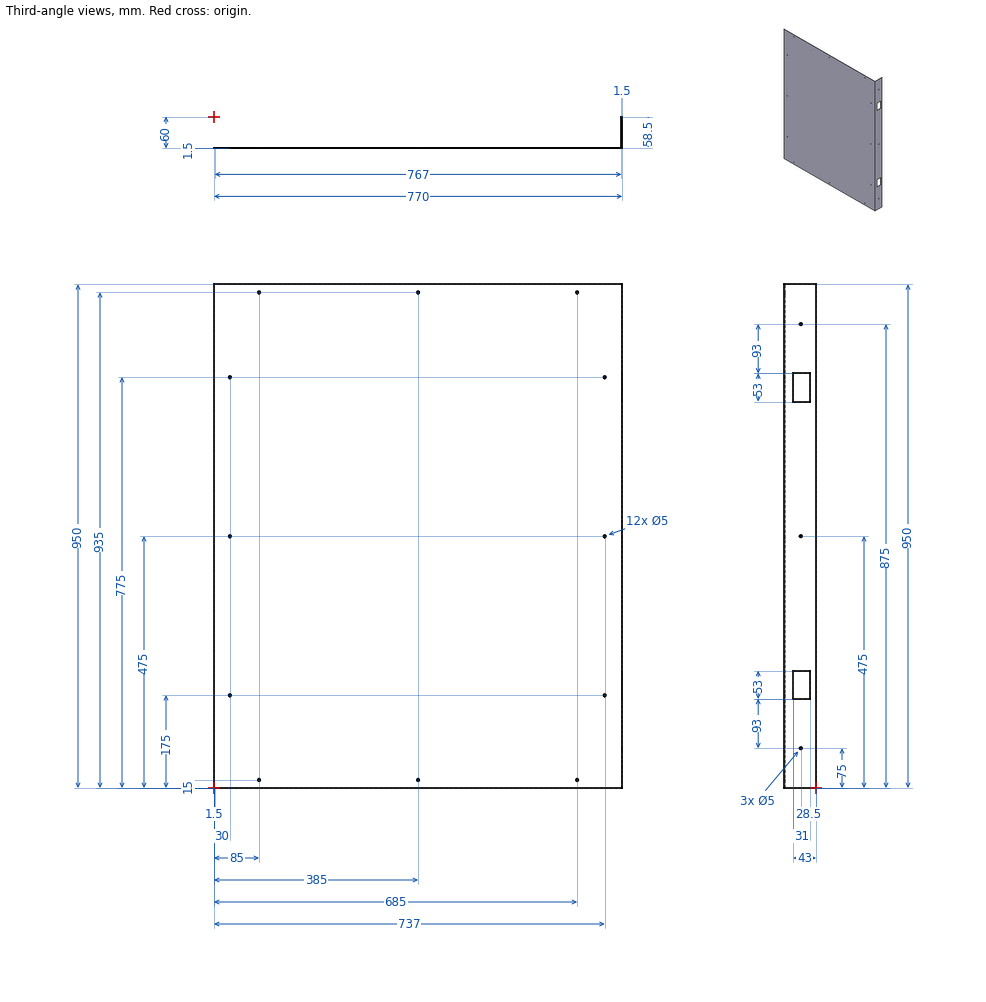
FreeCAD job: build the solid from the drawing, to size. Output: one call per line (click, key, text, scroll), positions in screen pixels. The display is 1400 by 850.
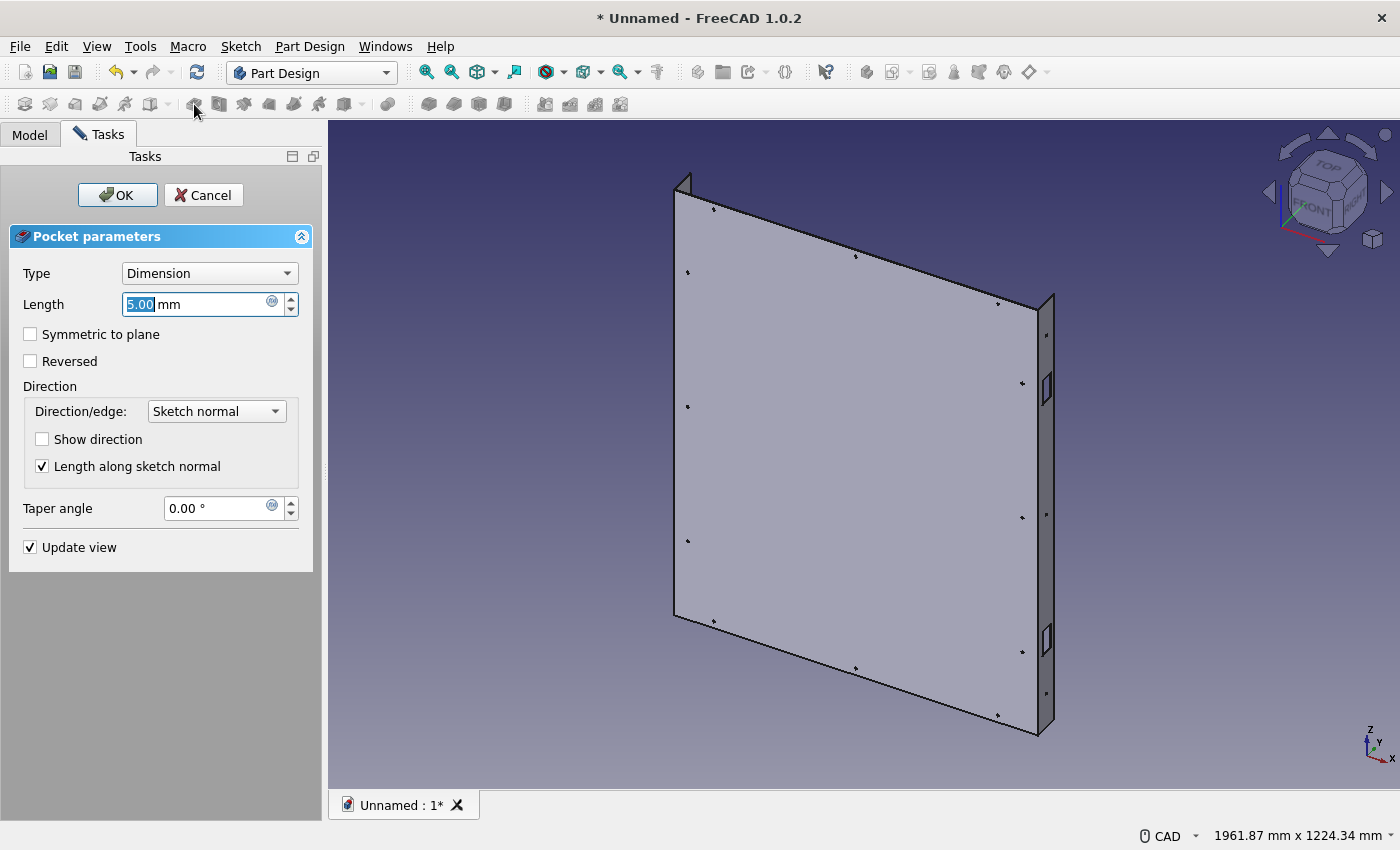
text(1.5)
key(Tab)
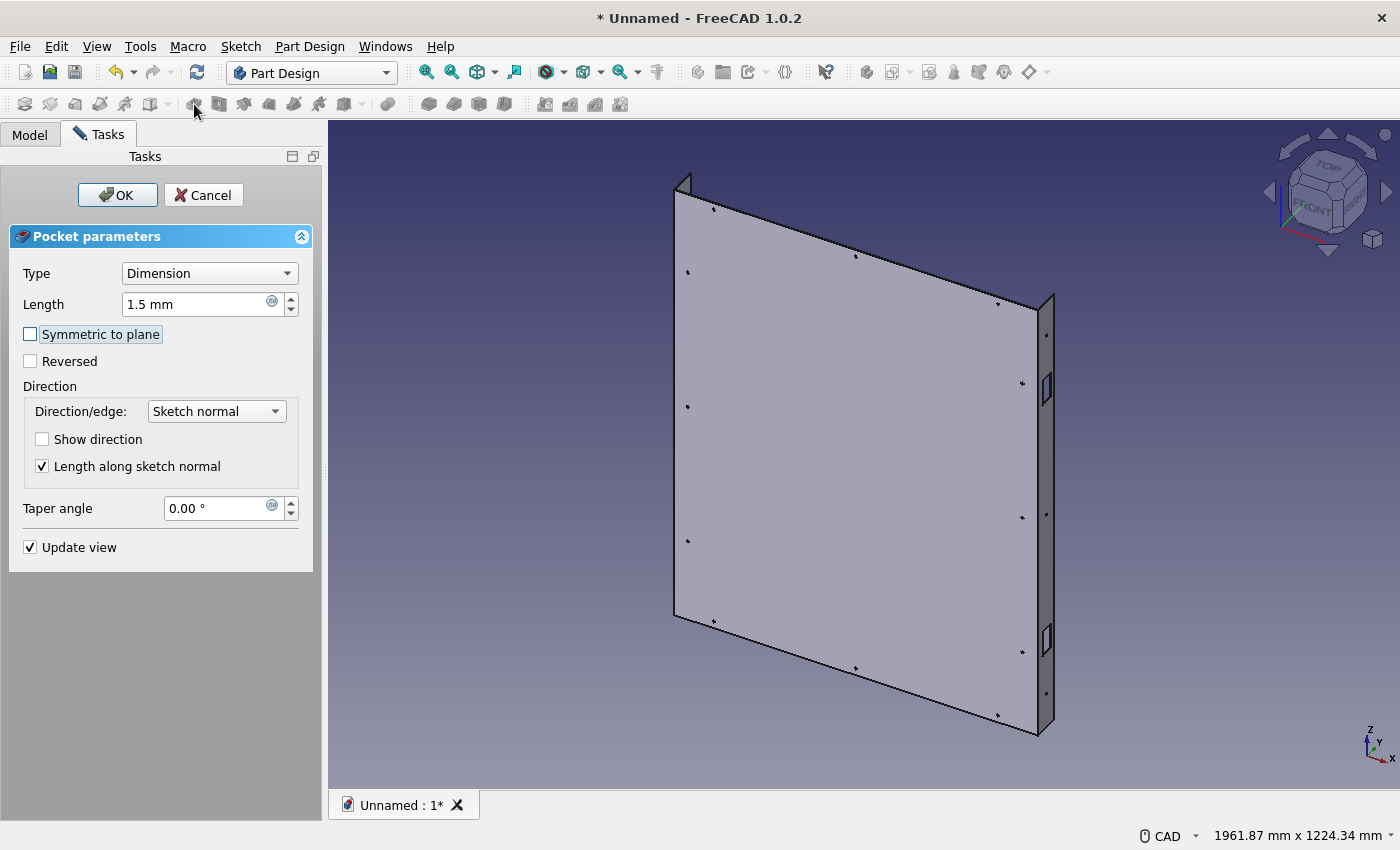
click(118, 195)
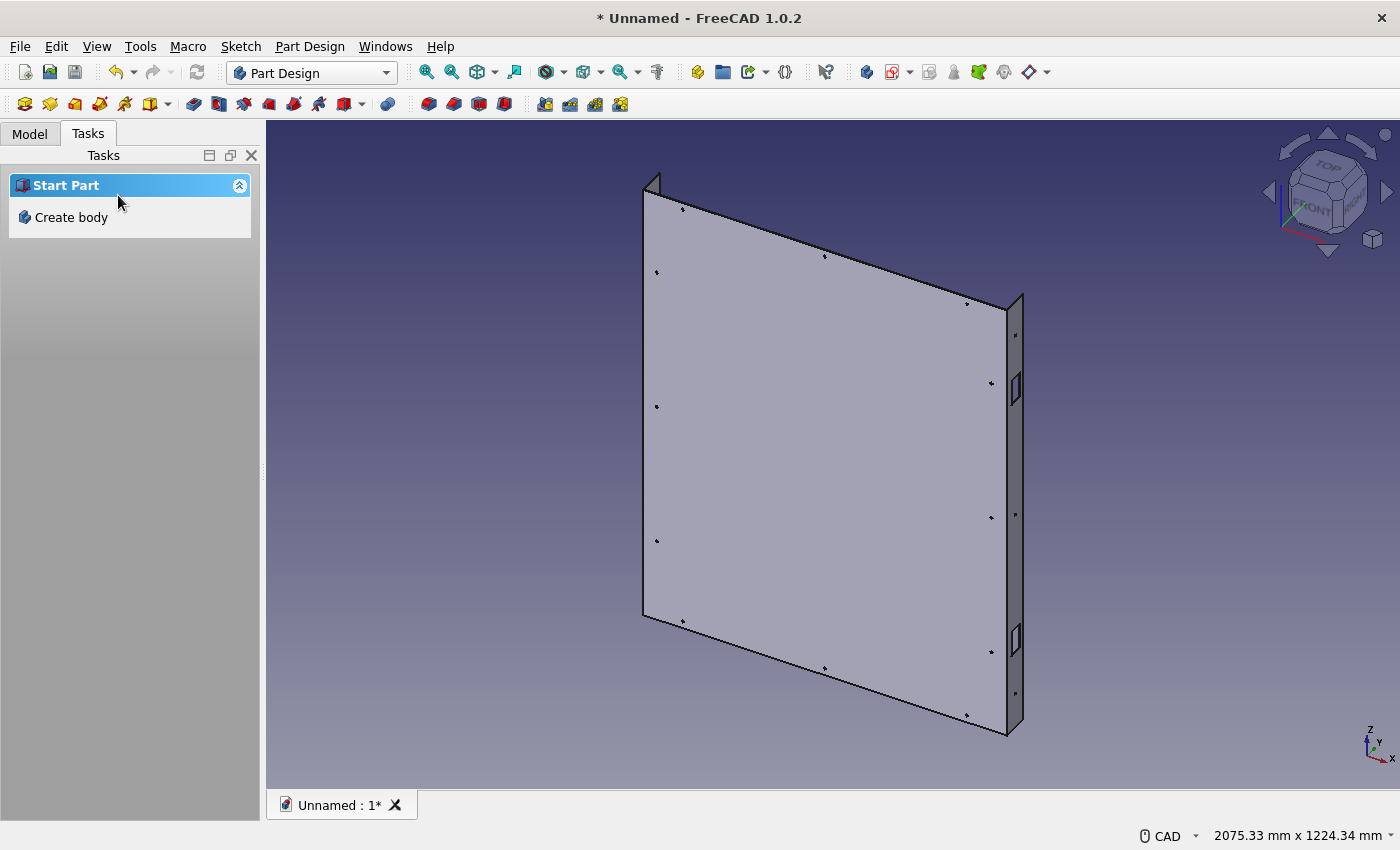
click(892, 72)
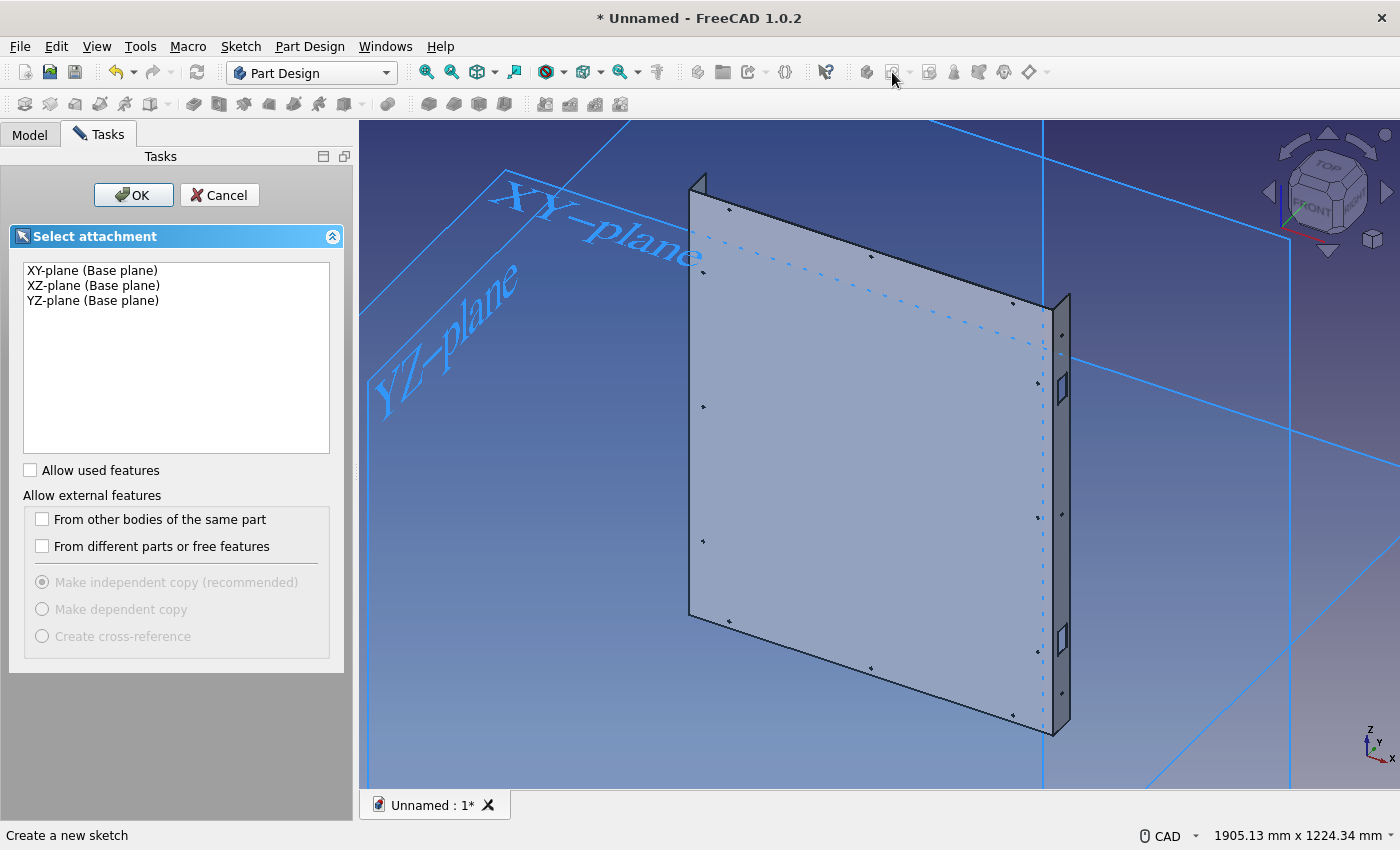
click(84, 286)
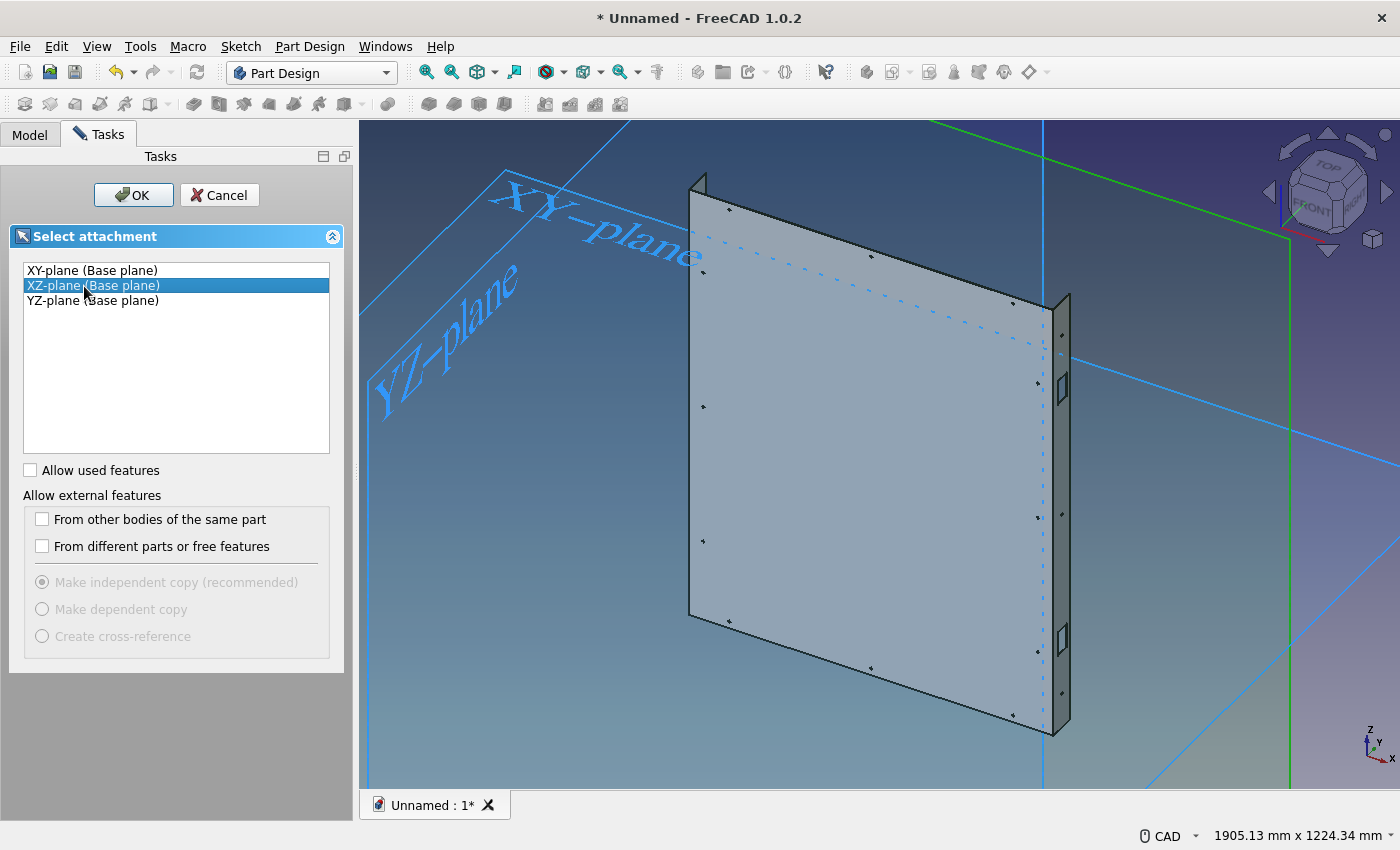
click(134, 195)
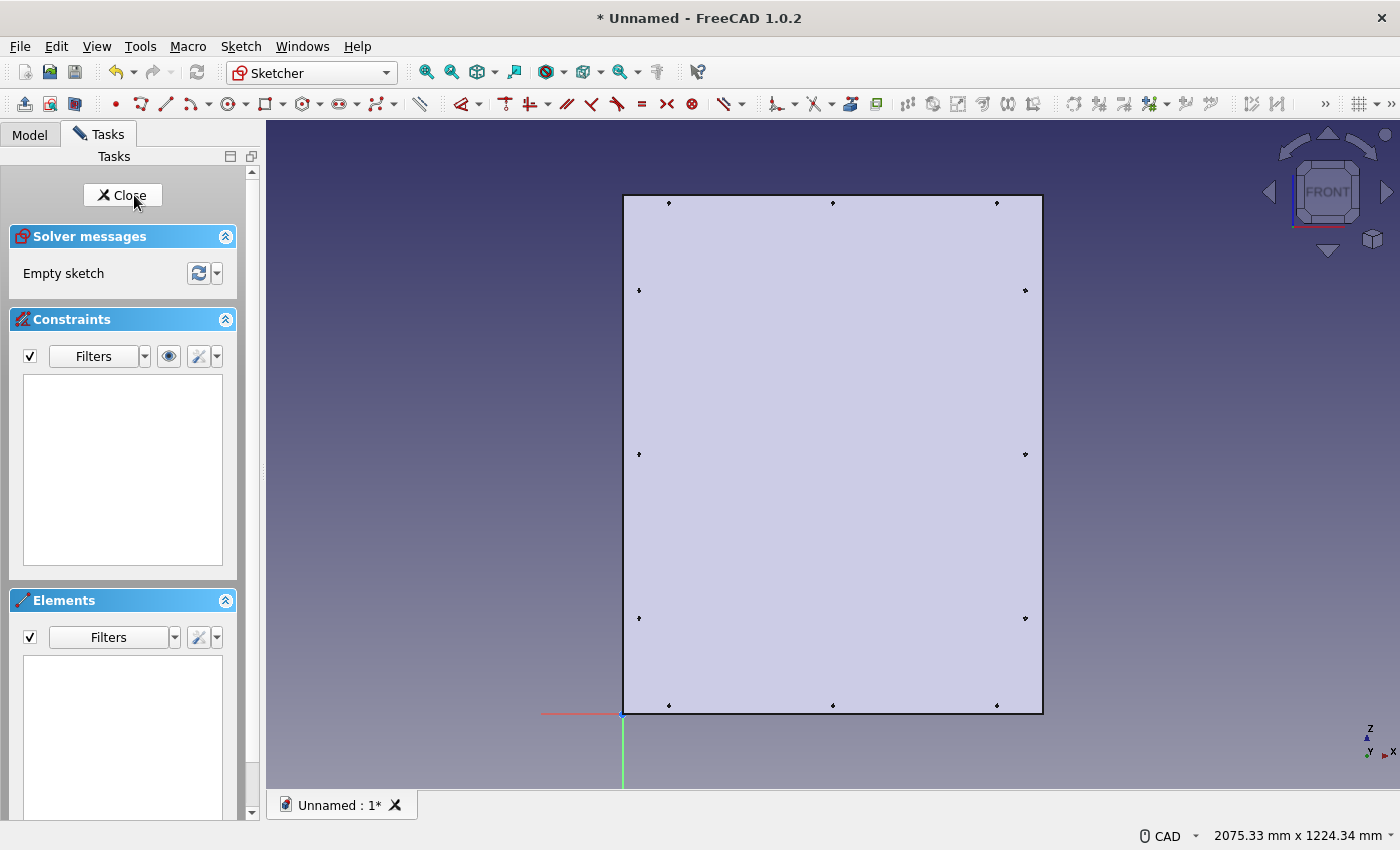
click(75, 104)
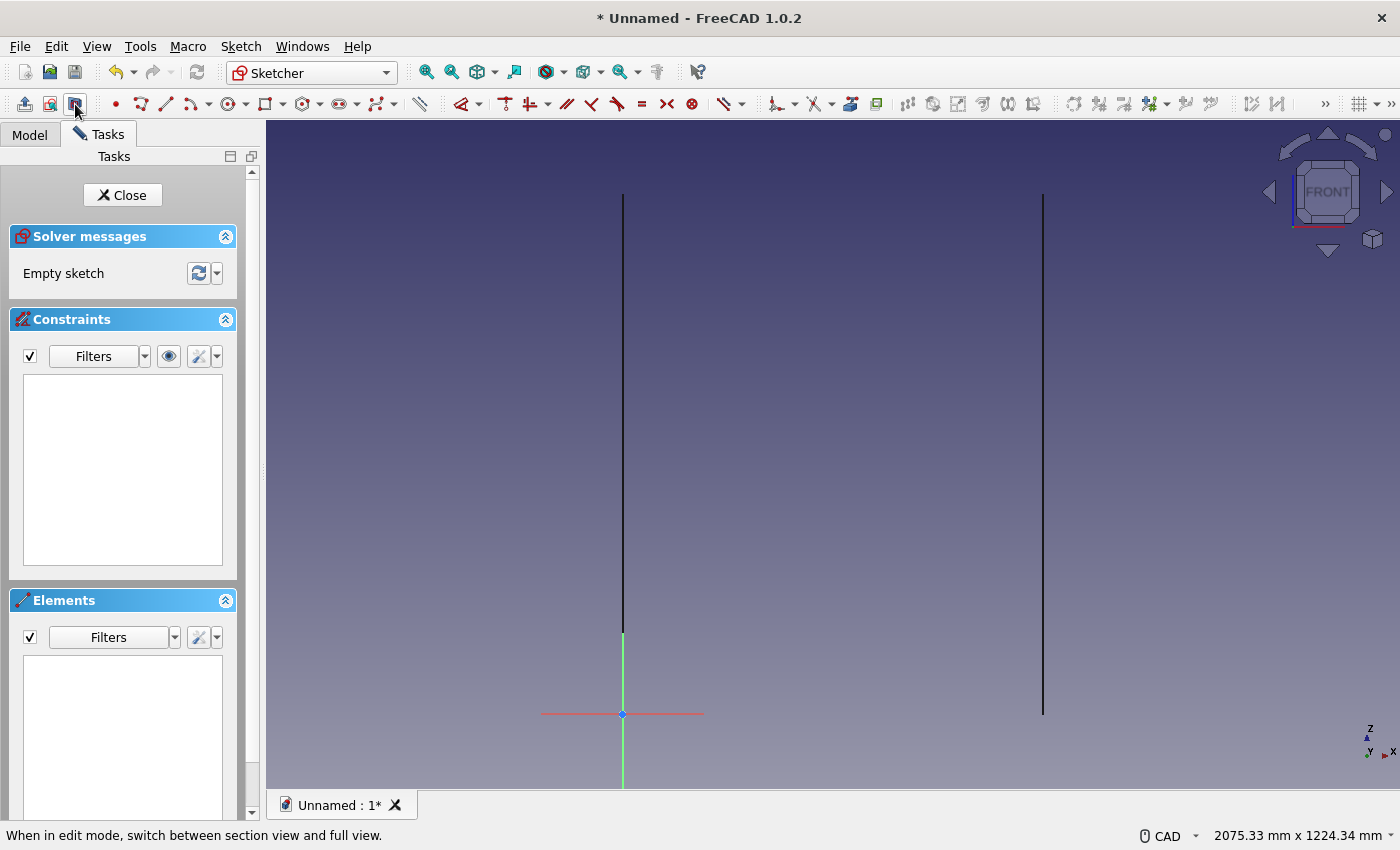
click(264, 104)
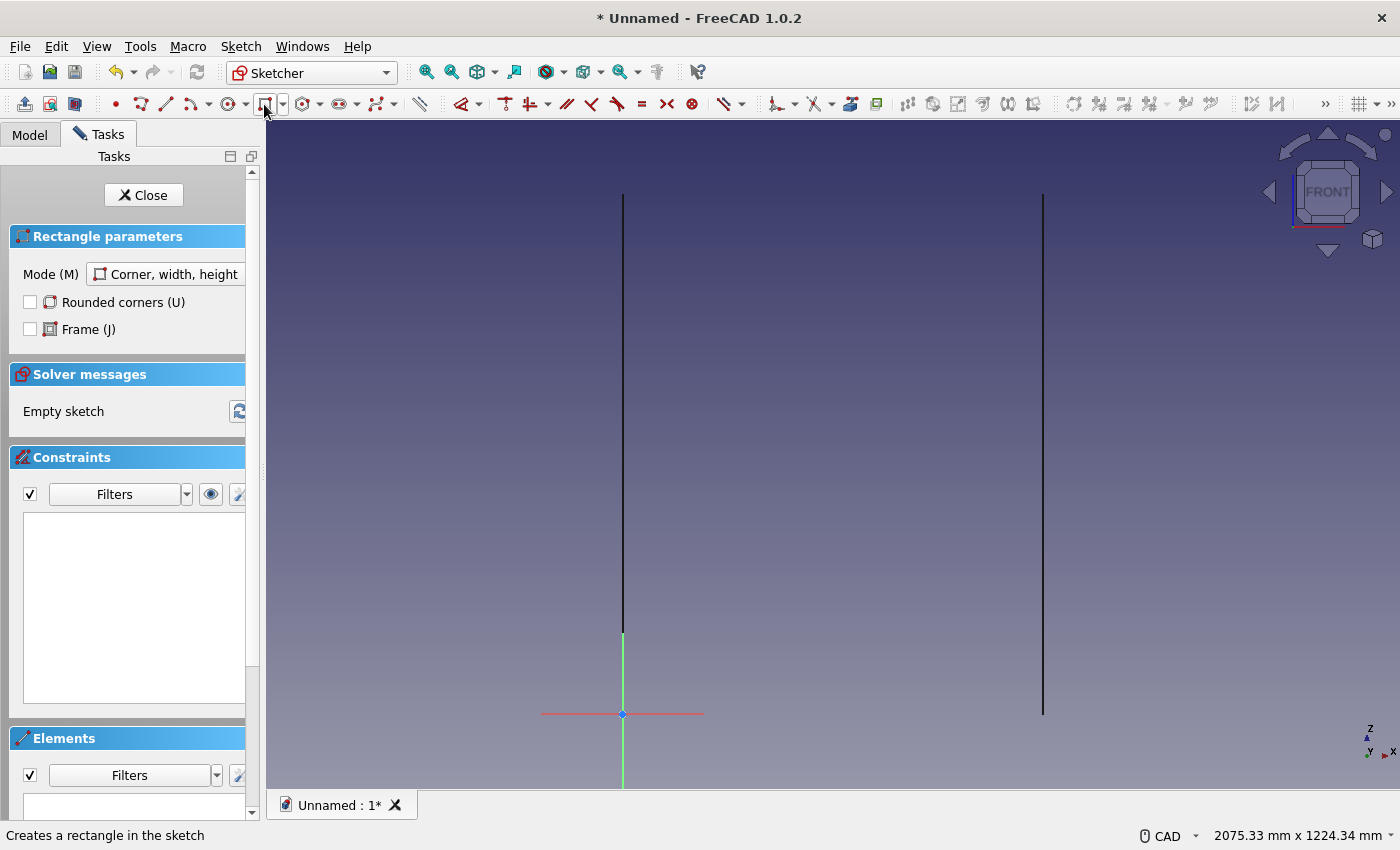
scroll(623, 714, up, 15)